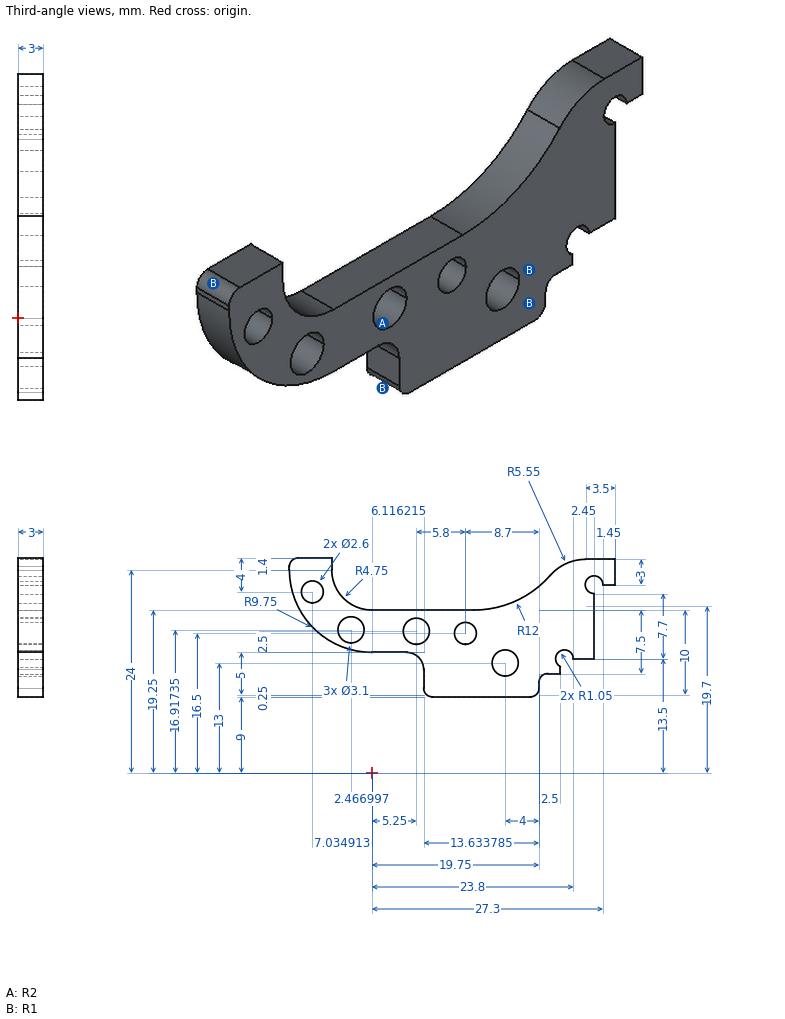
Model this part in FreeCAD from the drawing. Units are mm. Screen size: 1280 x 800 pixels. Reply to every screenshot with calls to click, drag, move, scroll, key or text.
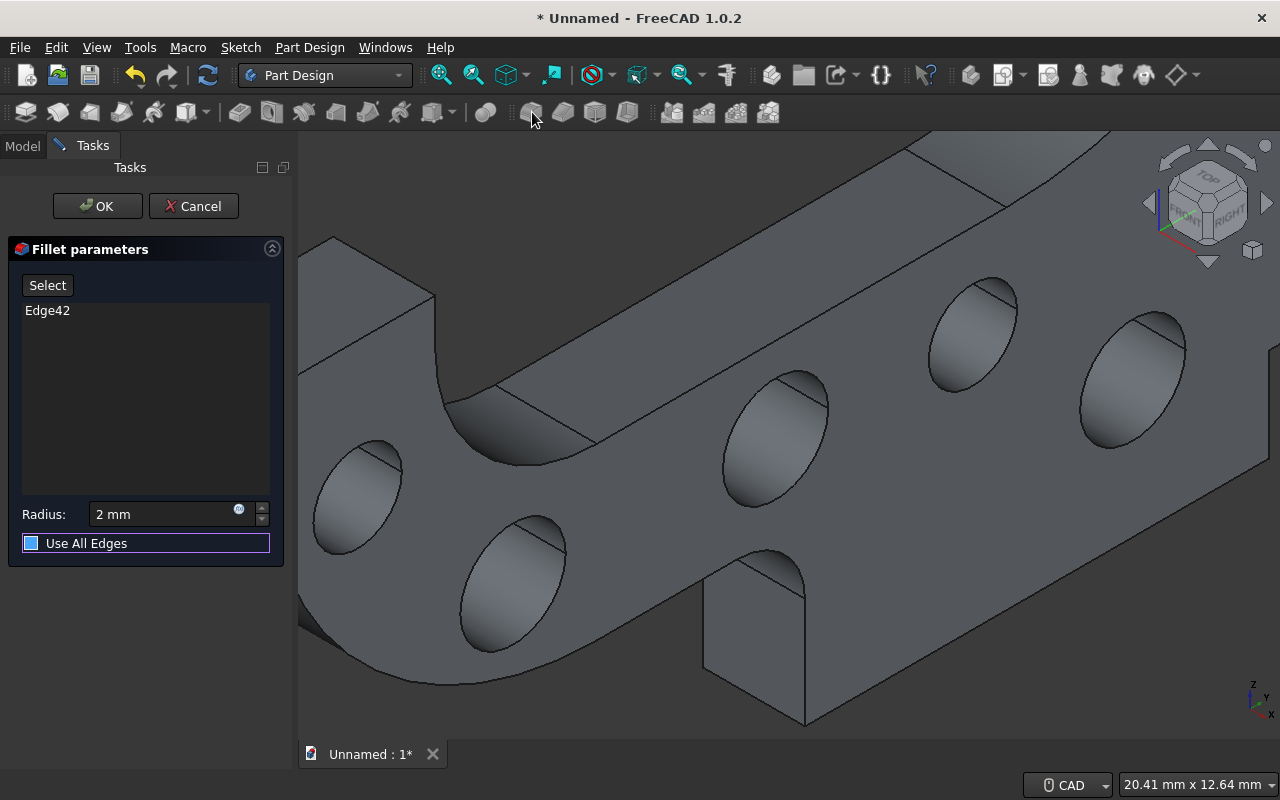
click(98, 206)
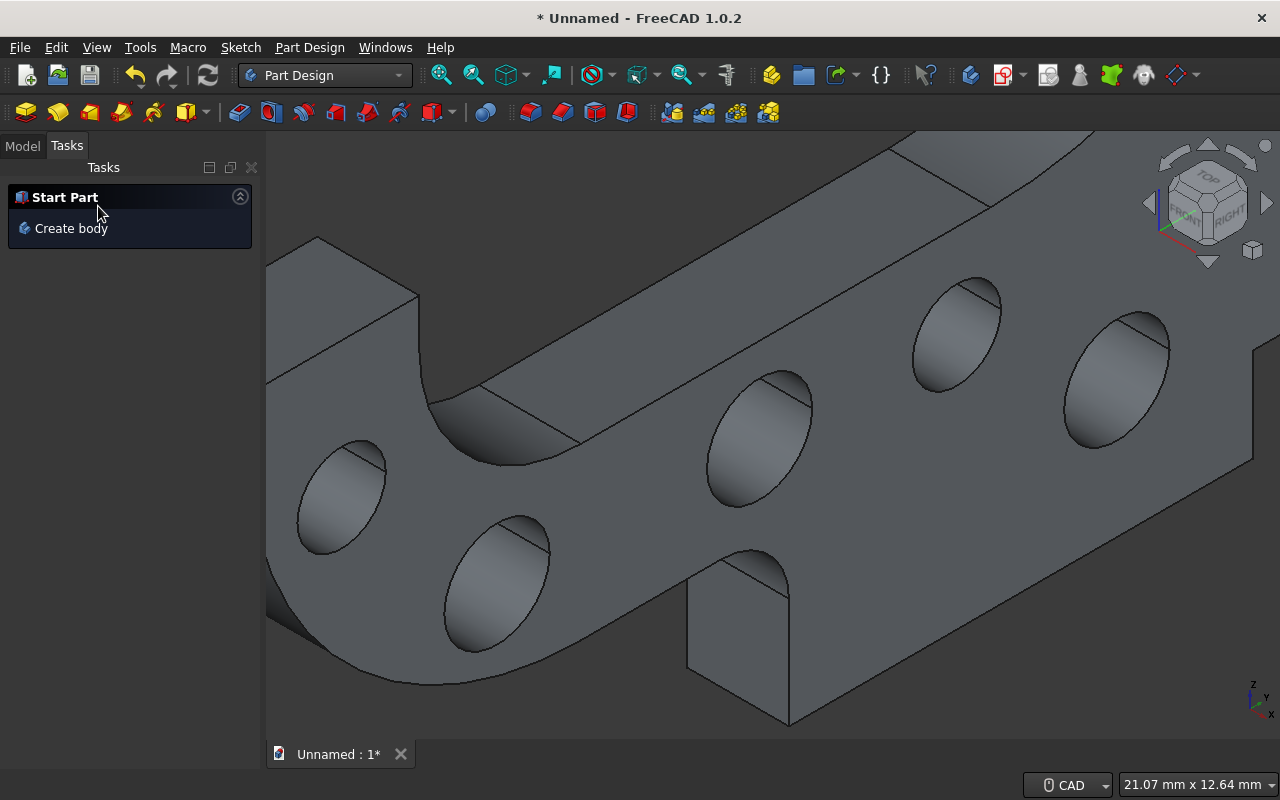
key(v)
key(f)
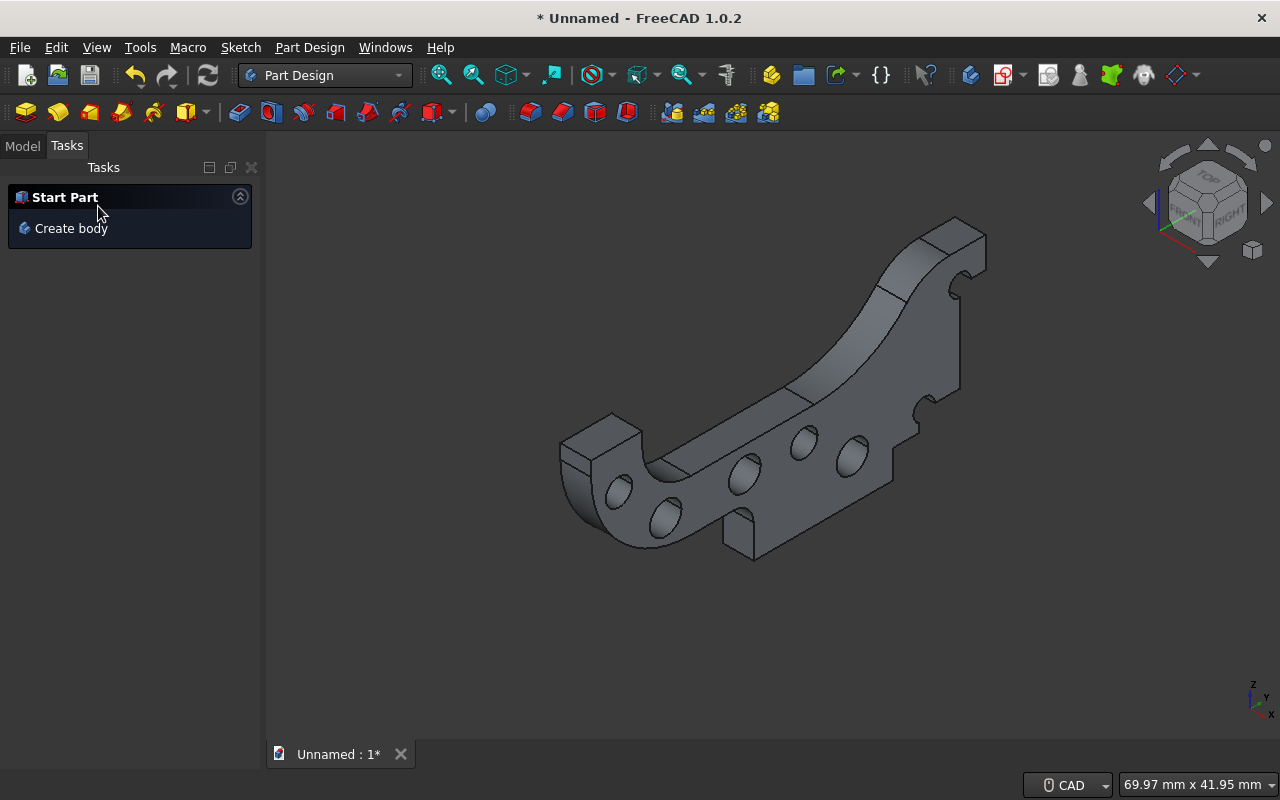
click(576, 451)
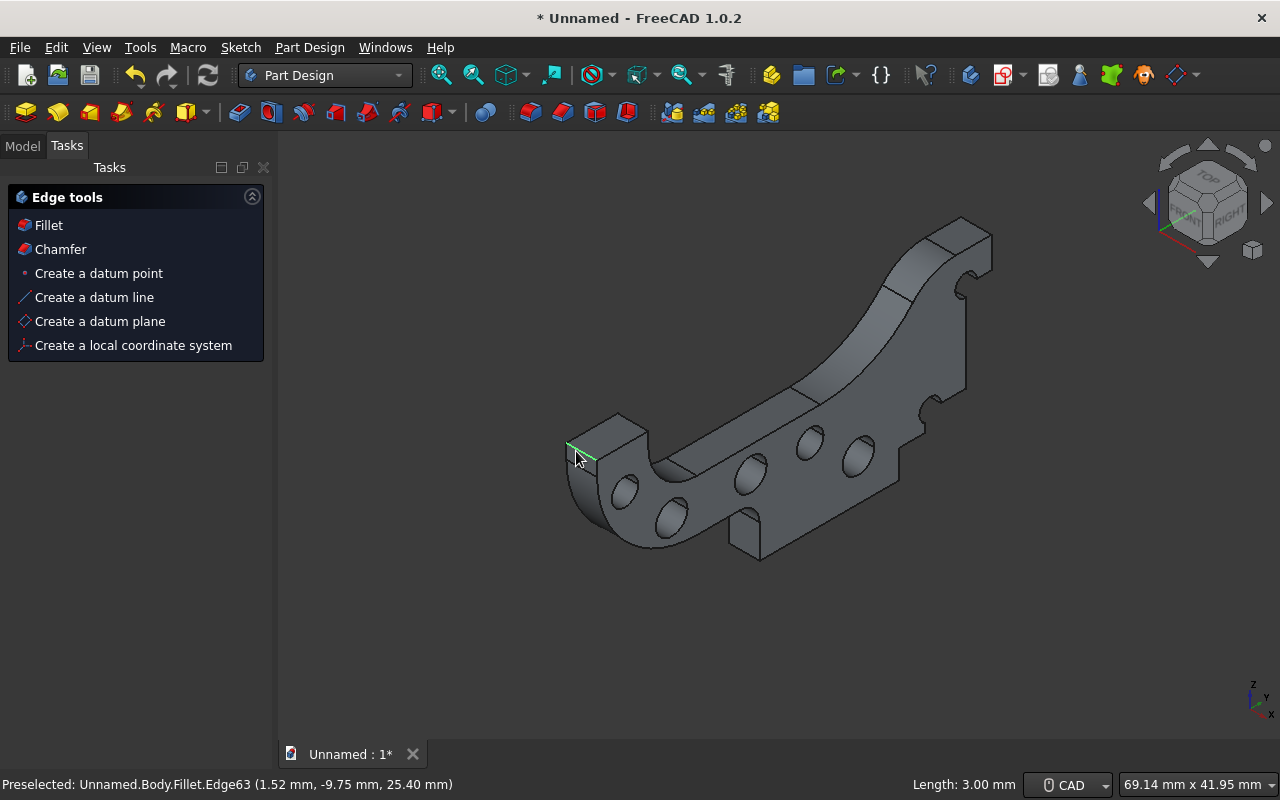
key(2)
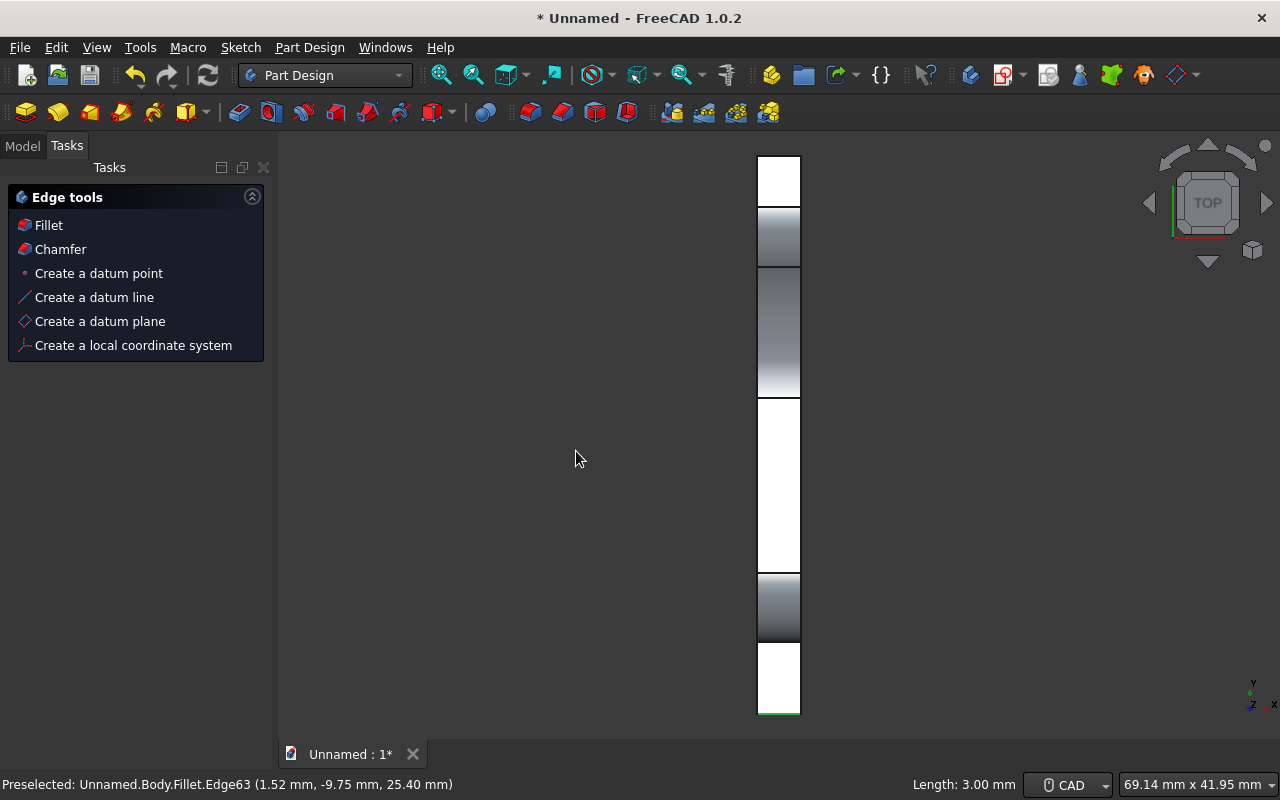
key(0)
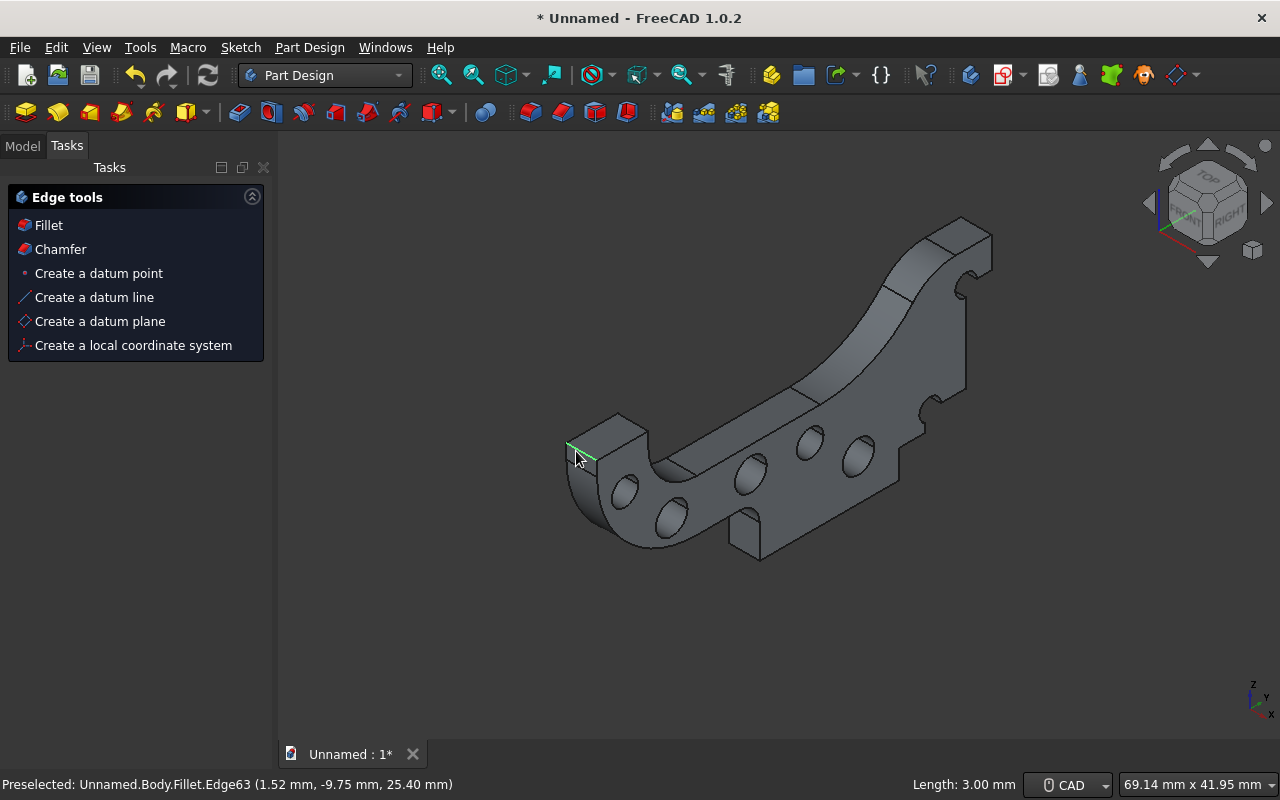
key(1)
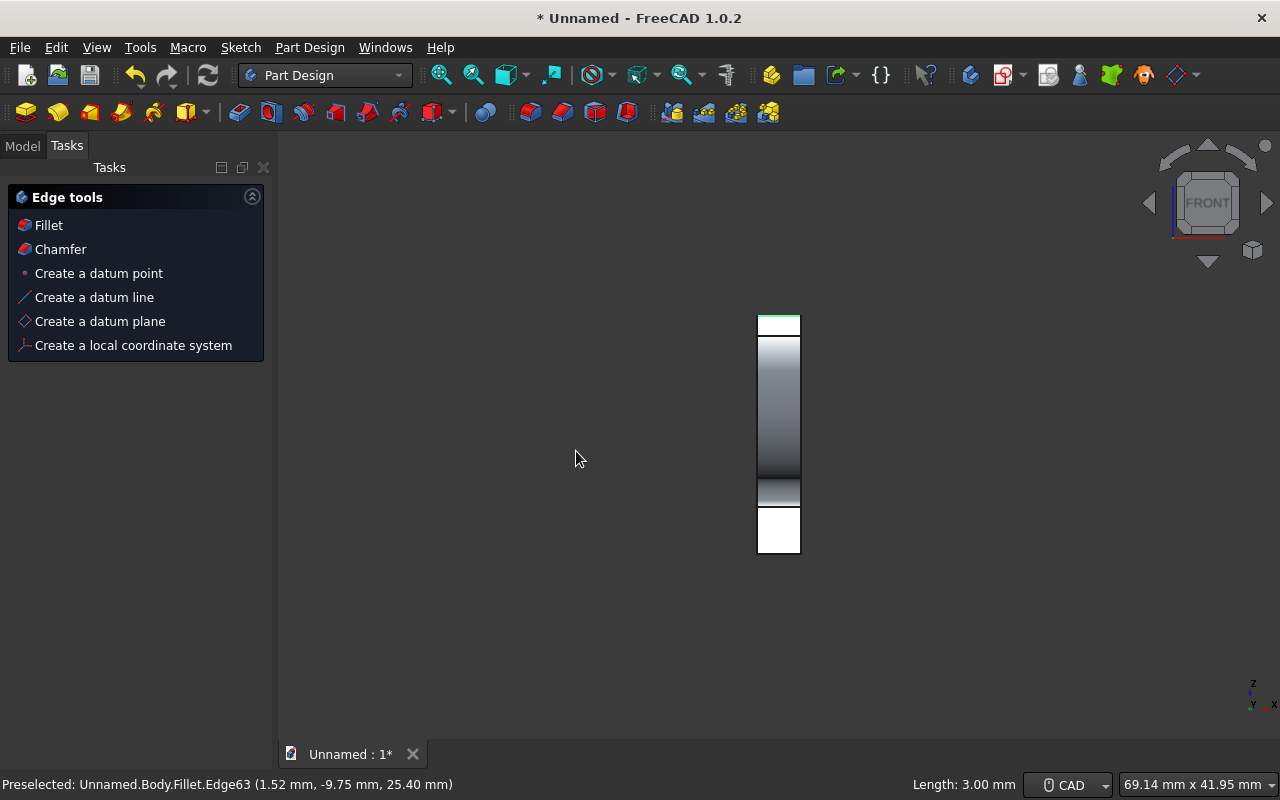
click(442, 76)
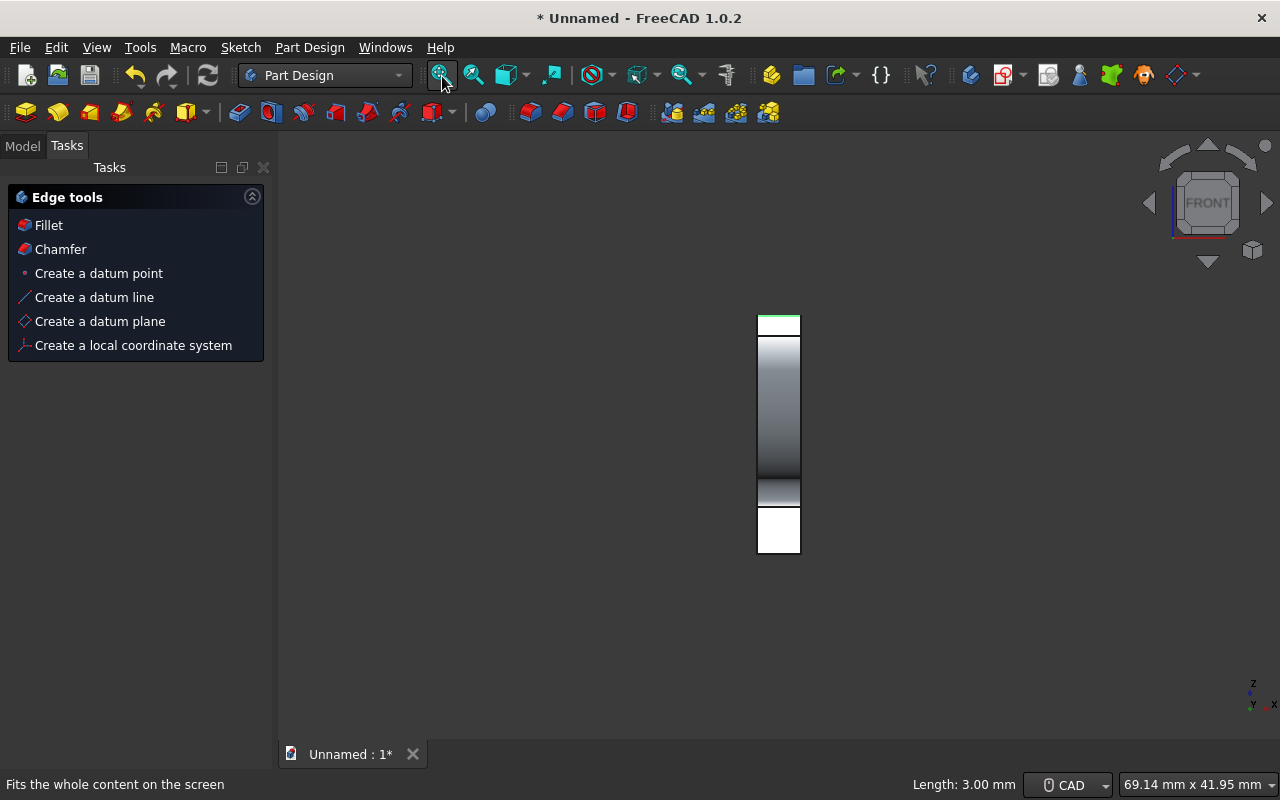
click(779, 553, ctrl)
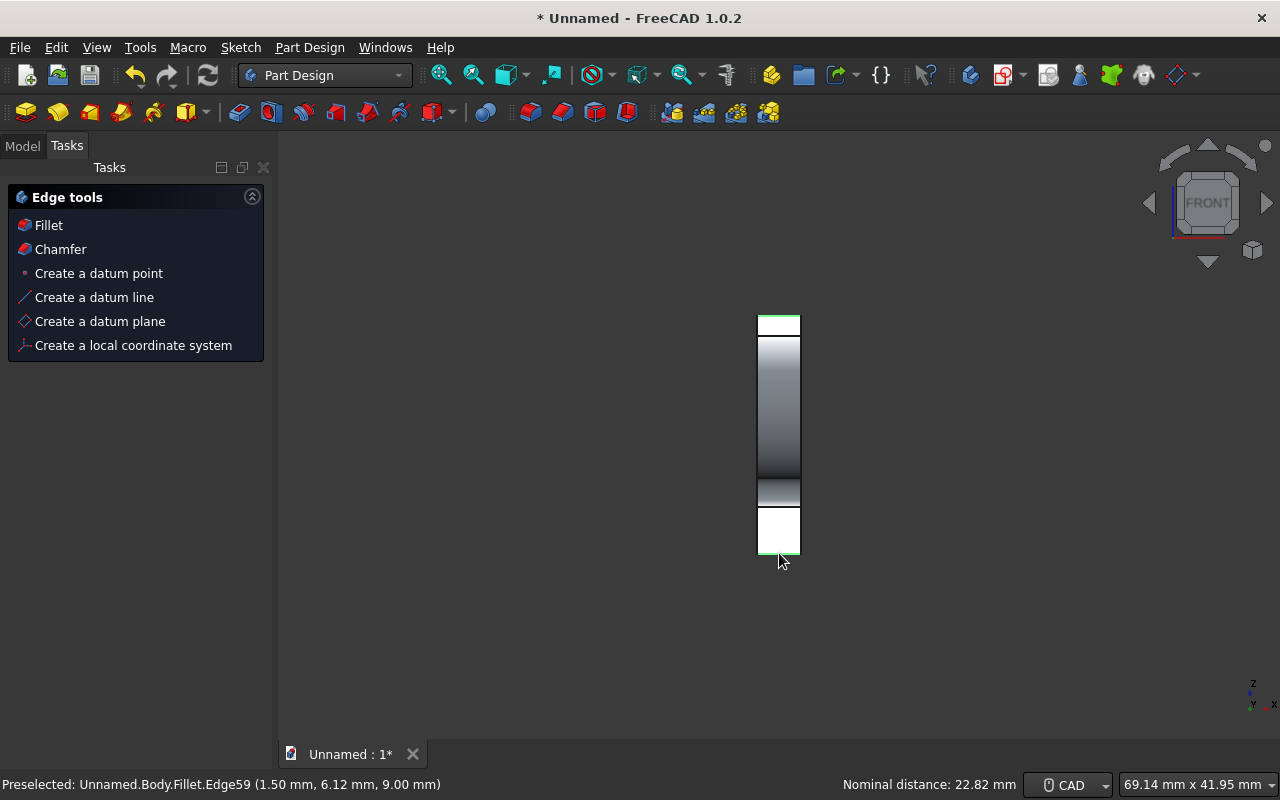
key(3)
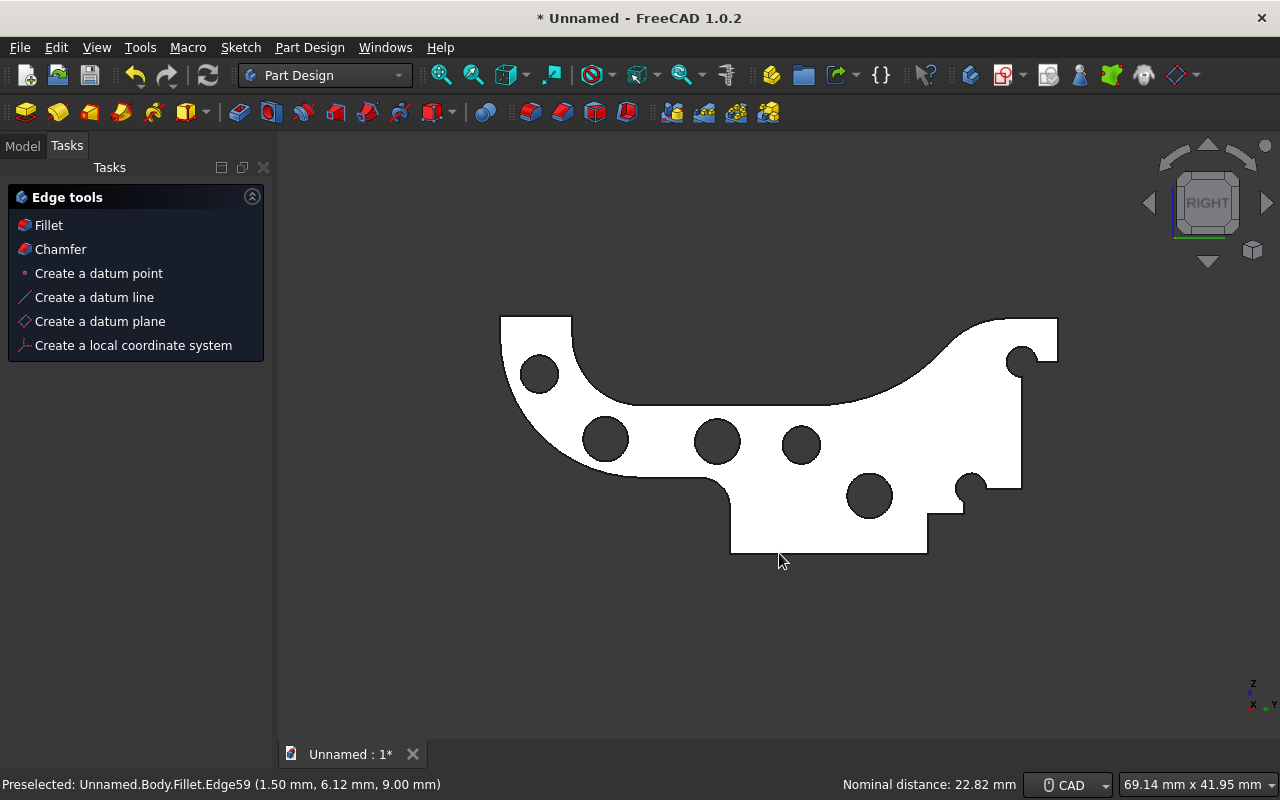
key(5)